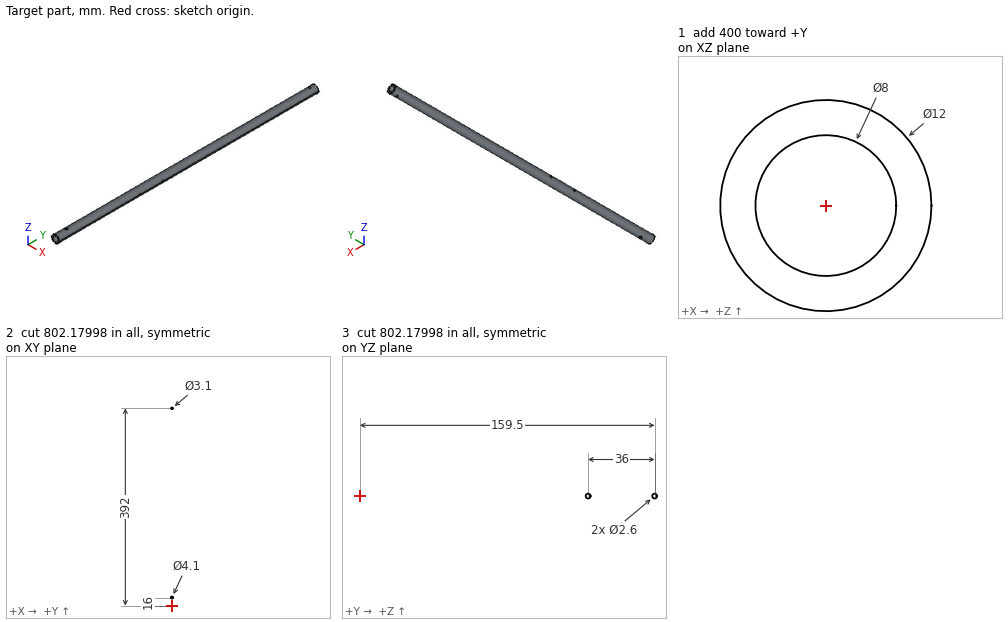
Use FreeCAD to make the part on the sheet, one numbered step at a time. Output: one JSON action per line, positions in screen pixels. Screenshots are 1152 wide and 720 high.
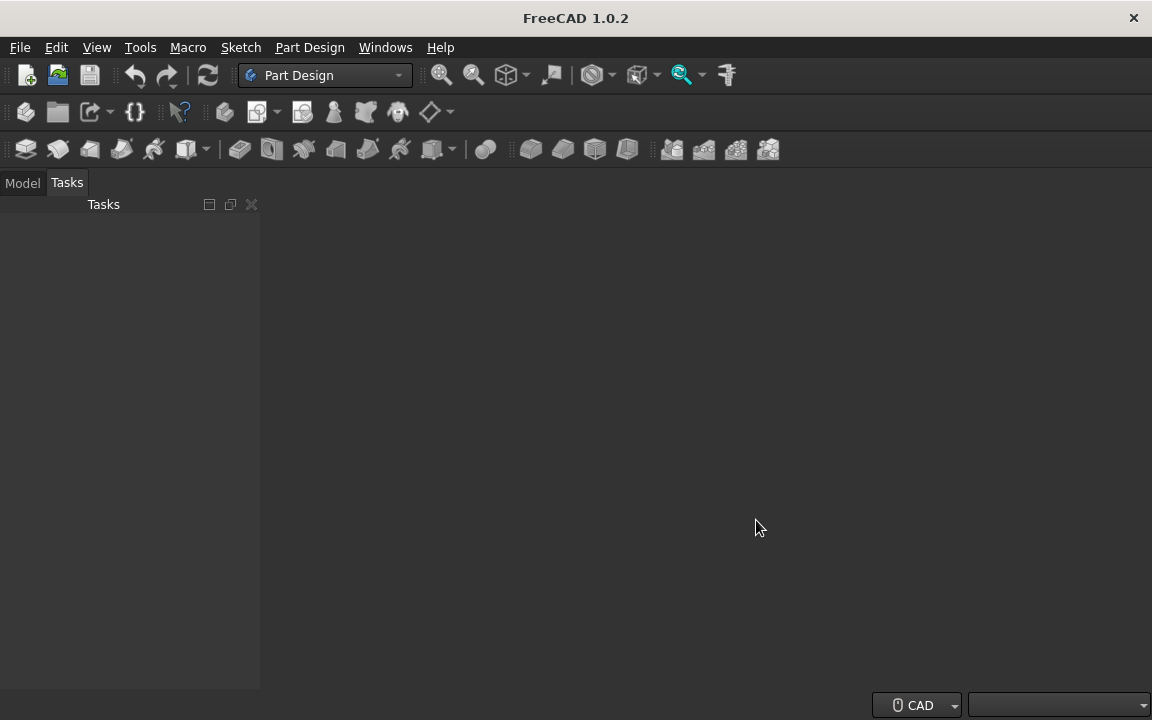
{"action": "left_click", "coordinate": [26, 76]}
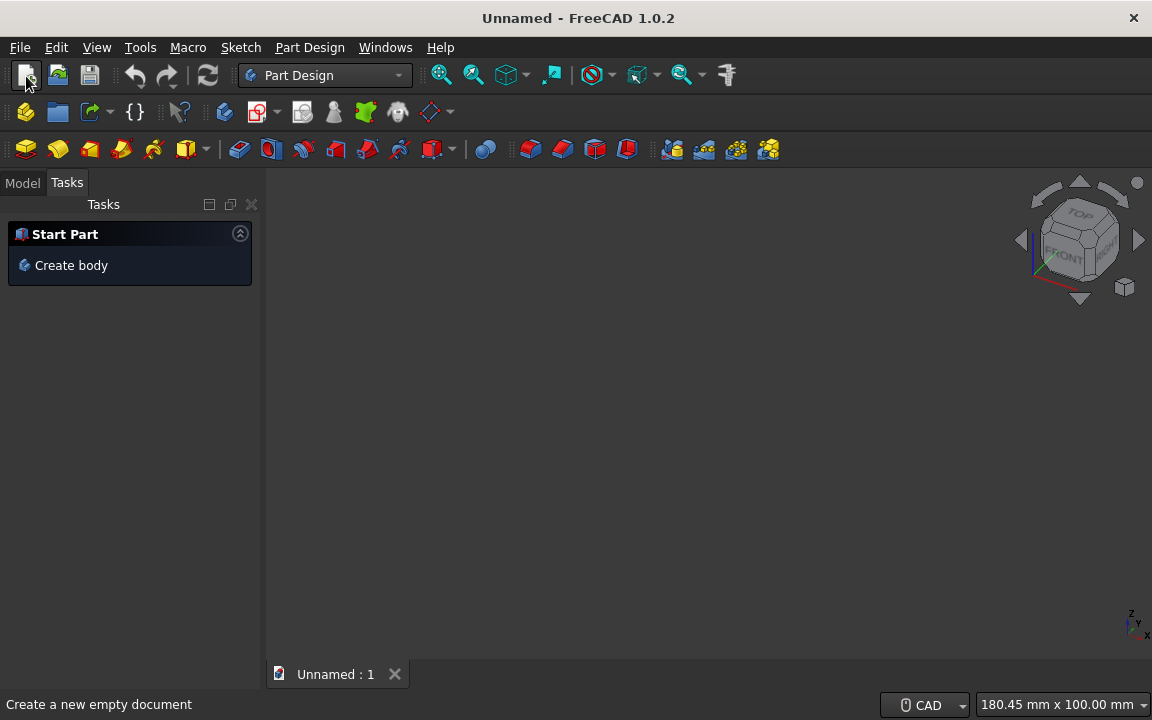
{"action": "left_click", "coordinate": [258, 112]}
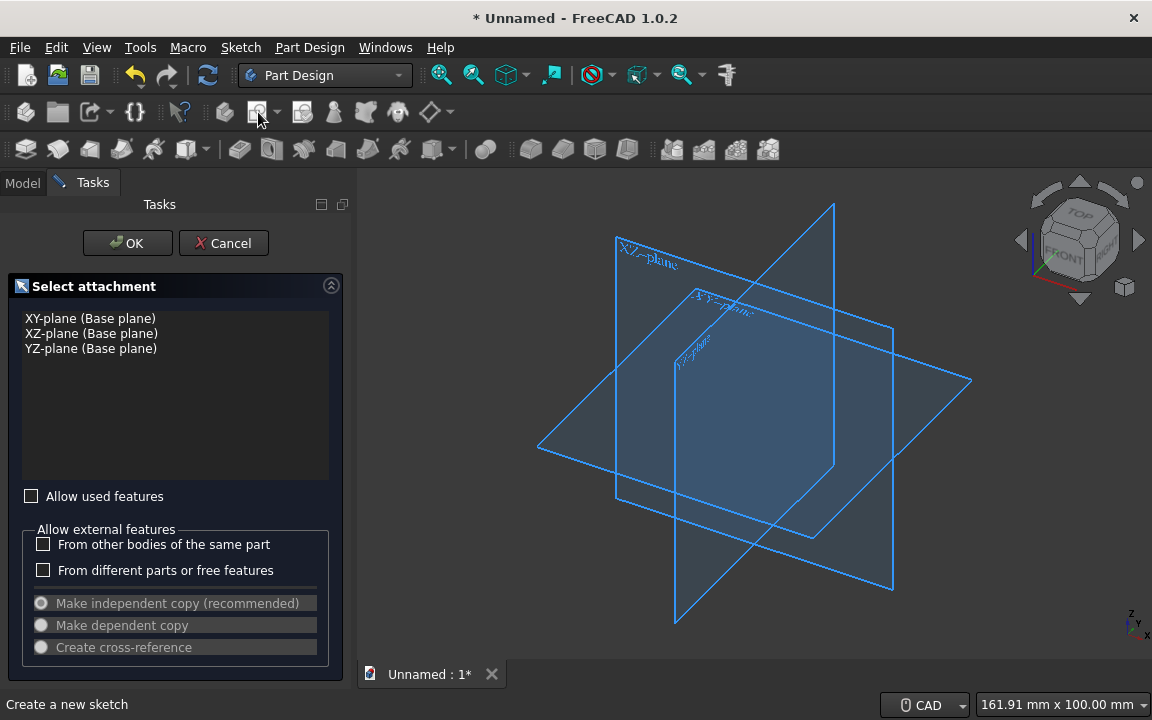
{"action": "left_click", "coordinate": [82, 334]}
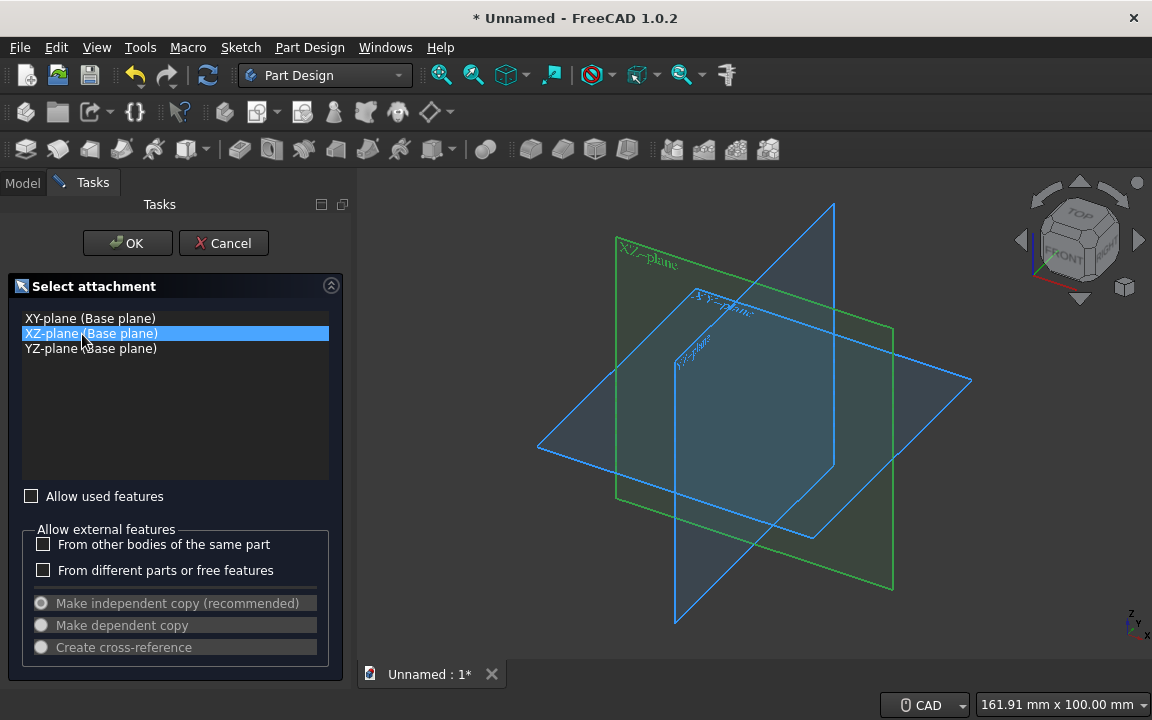
{"action": "left_click", "coordinate": [128, 243]}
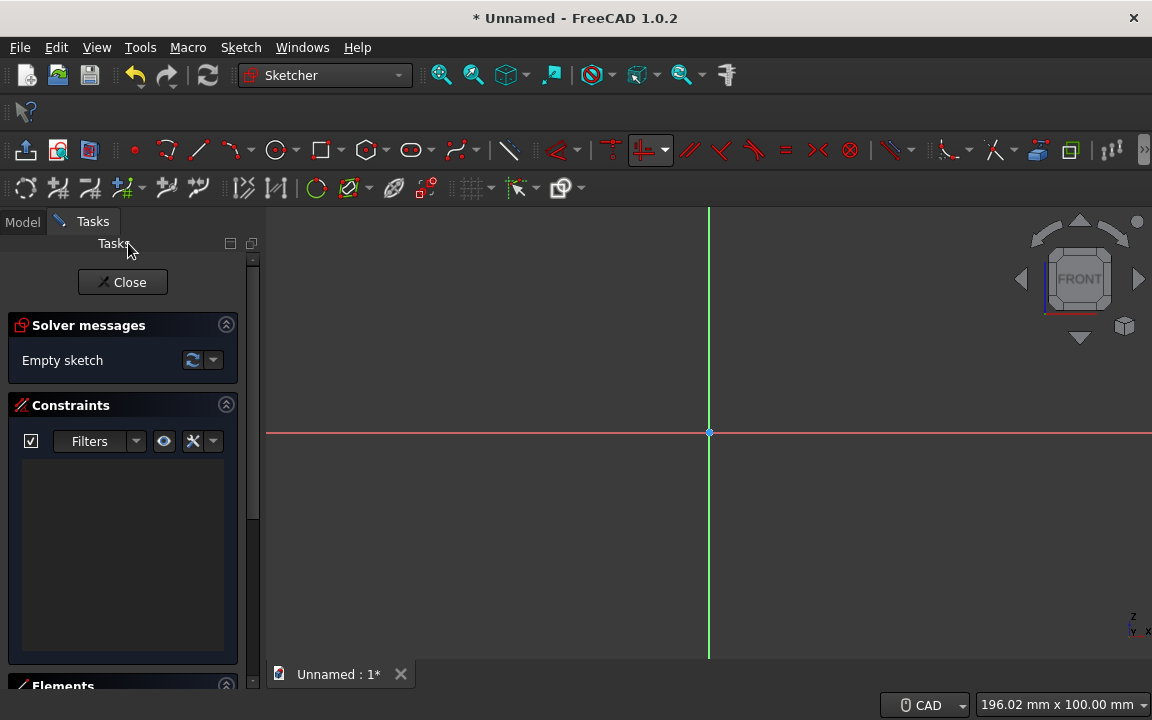
{"action": "scroll", "coordinate": [726, 433], "scroll_direction": "up", "scroll_amount": 8}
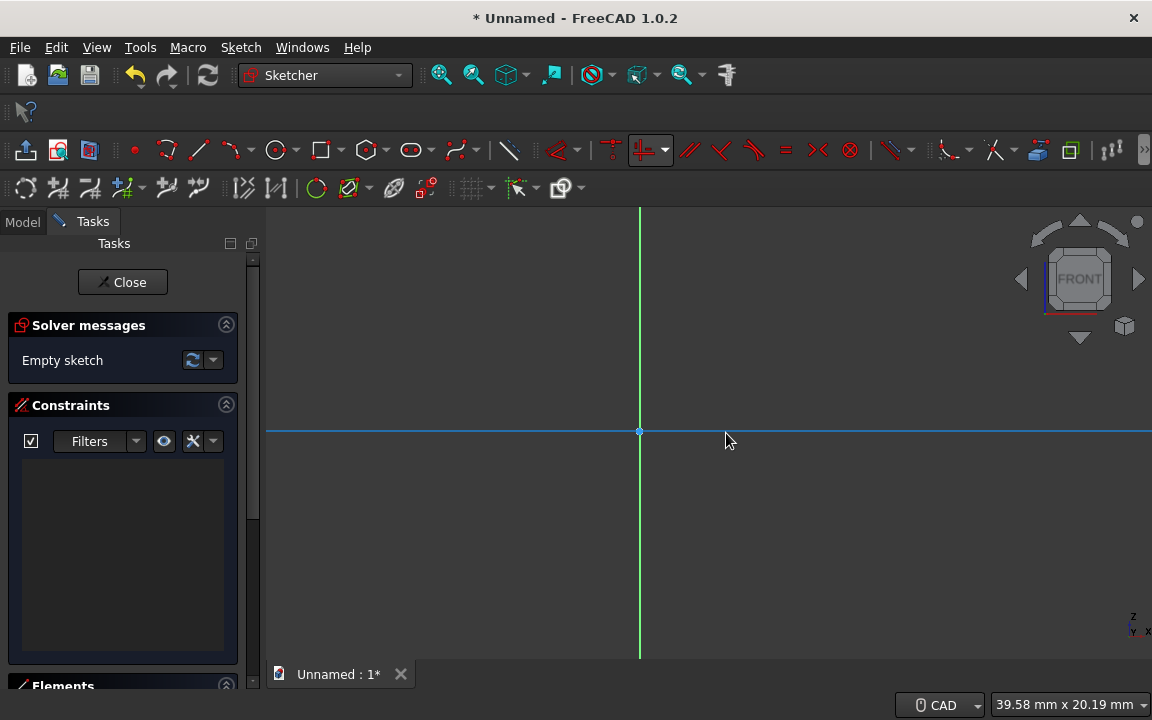
{"action": "key", "text": "g c"}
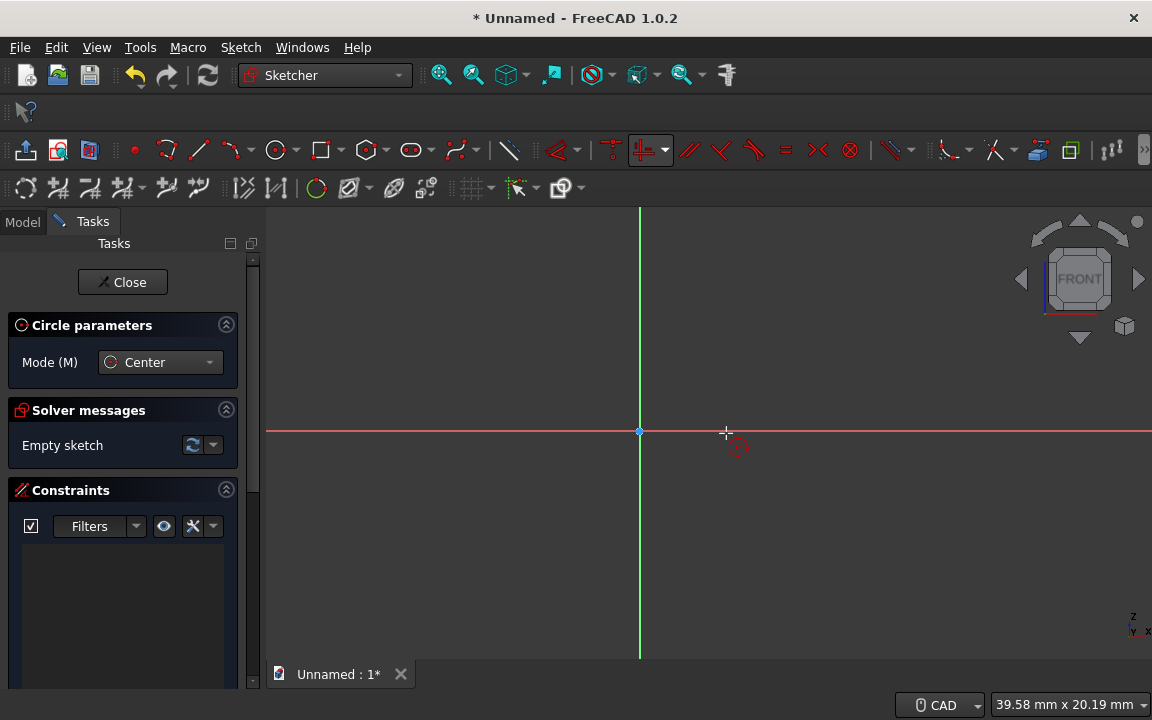
{"action": "left_click", "coordinate": [640, 431]}
{"action": "left_click", "coordinate": [735, 336]}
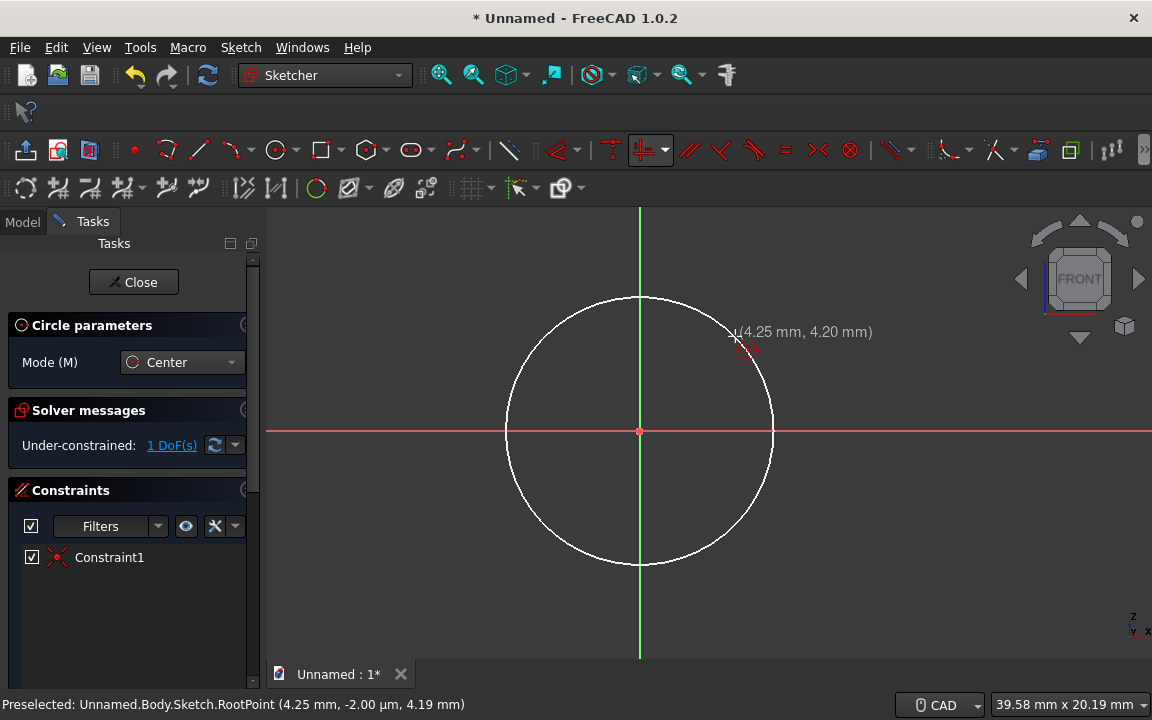
{"action": "left_click", "coordinate": [640, 431]}
{"action": "left_click", "coordinate": [703, 368]}
{"action": "key", "text": "Escape"}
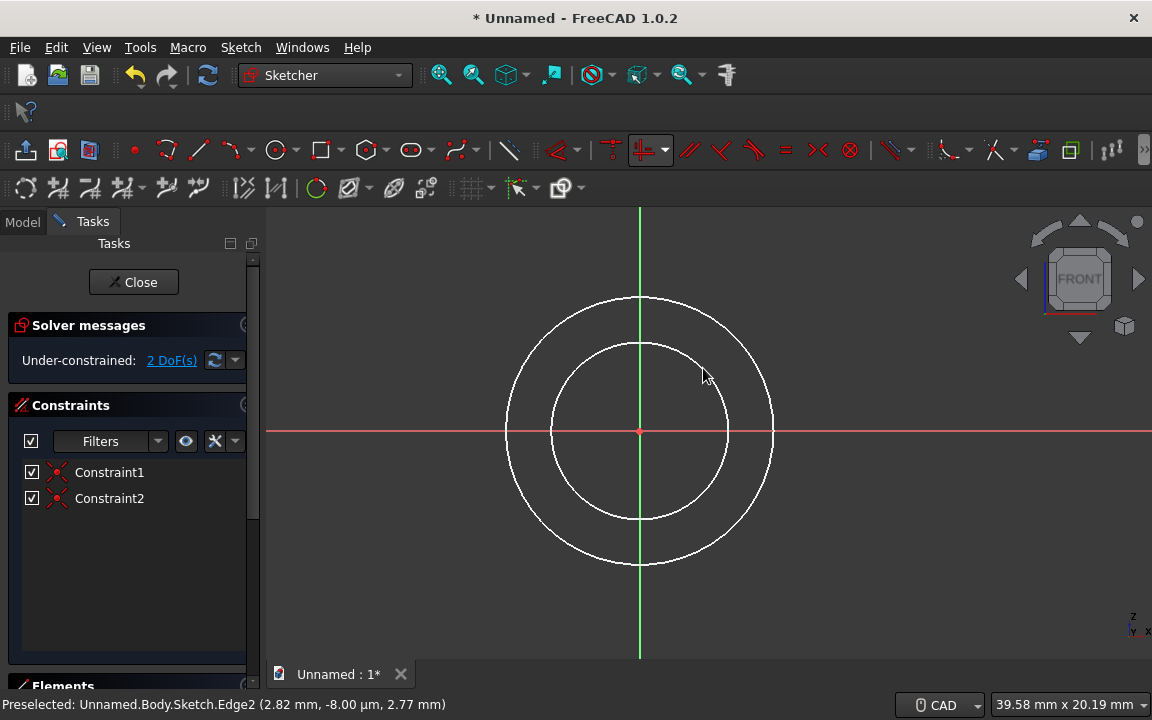
{"action": "key", "text": "d"}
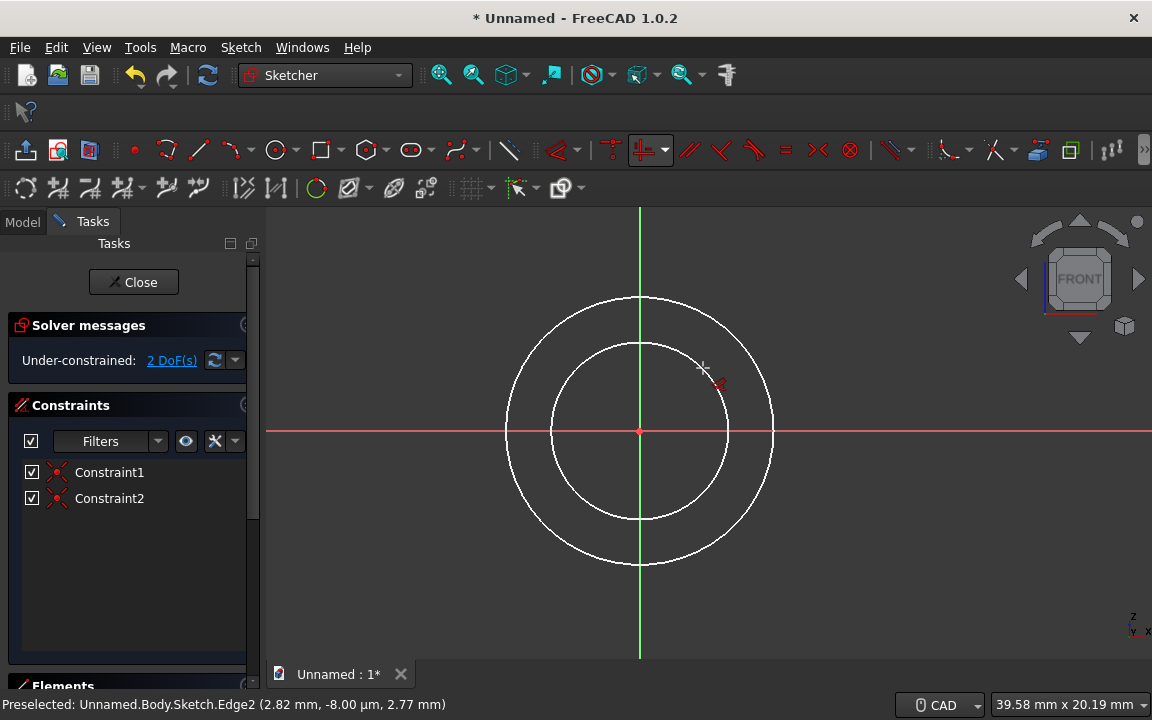
{"action": "left_click", "coordinate": [734, 336]}
{"action": "left_click", "coordinate": [757, 313]}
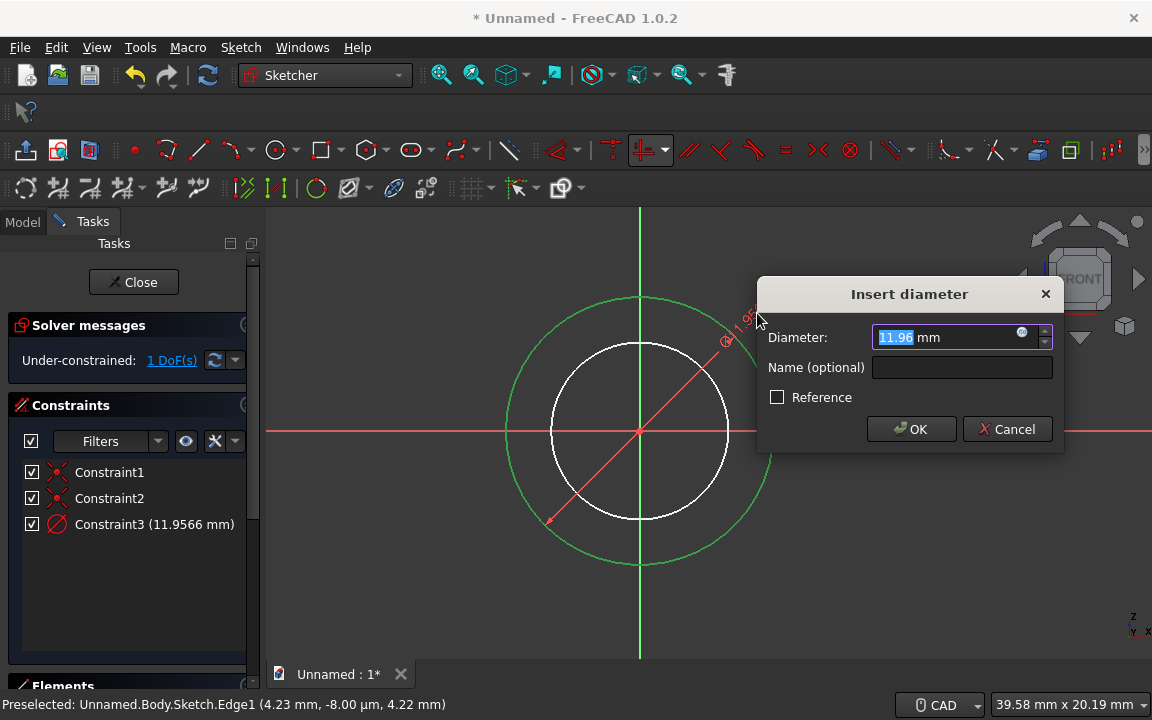
{"action": "type", "text": "12"}
{"action": "key", "text": "Return"}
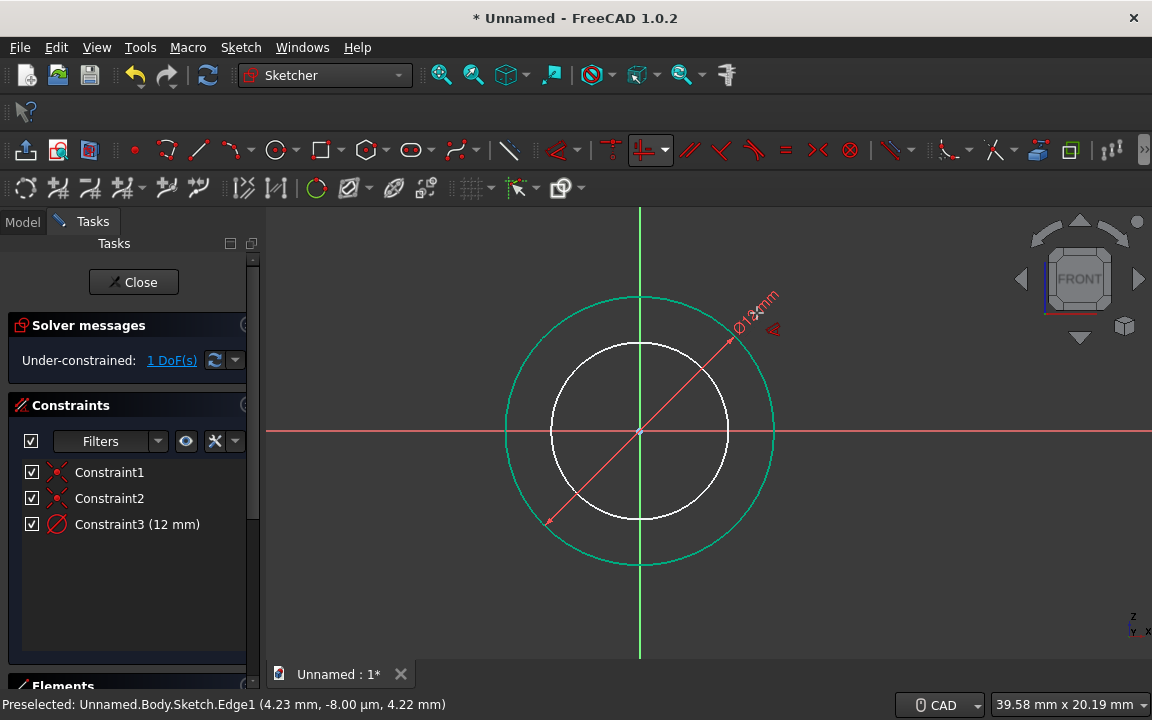
{"action": "left_click", "coordinate": [702, 368]}
{"action": "left_click", "coordinate": [724, 345]}